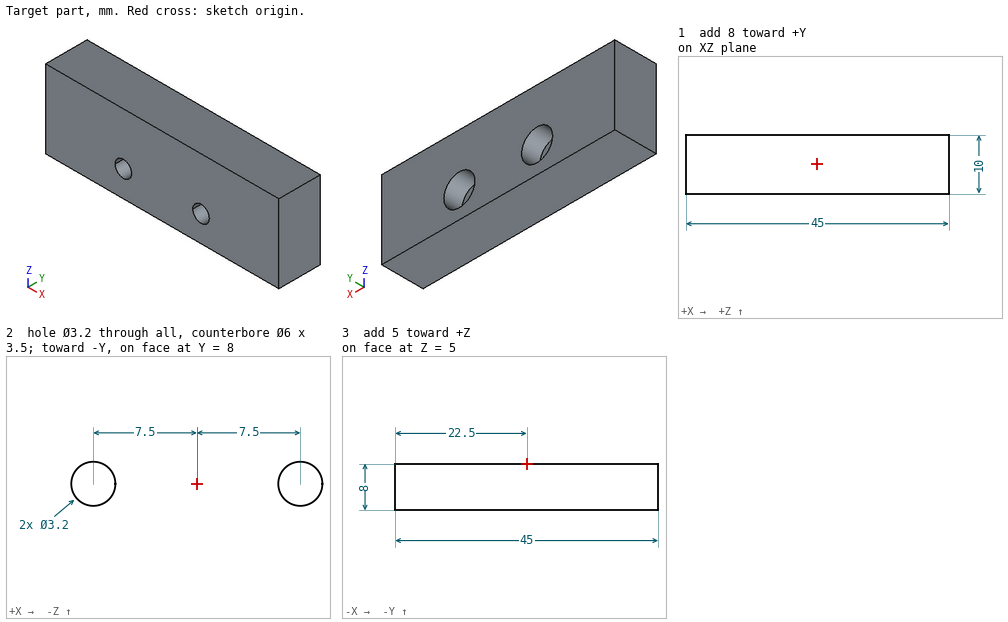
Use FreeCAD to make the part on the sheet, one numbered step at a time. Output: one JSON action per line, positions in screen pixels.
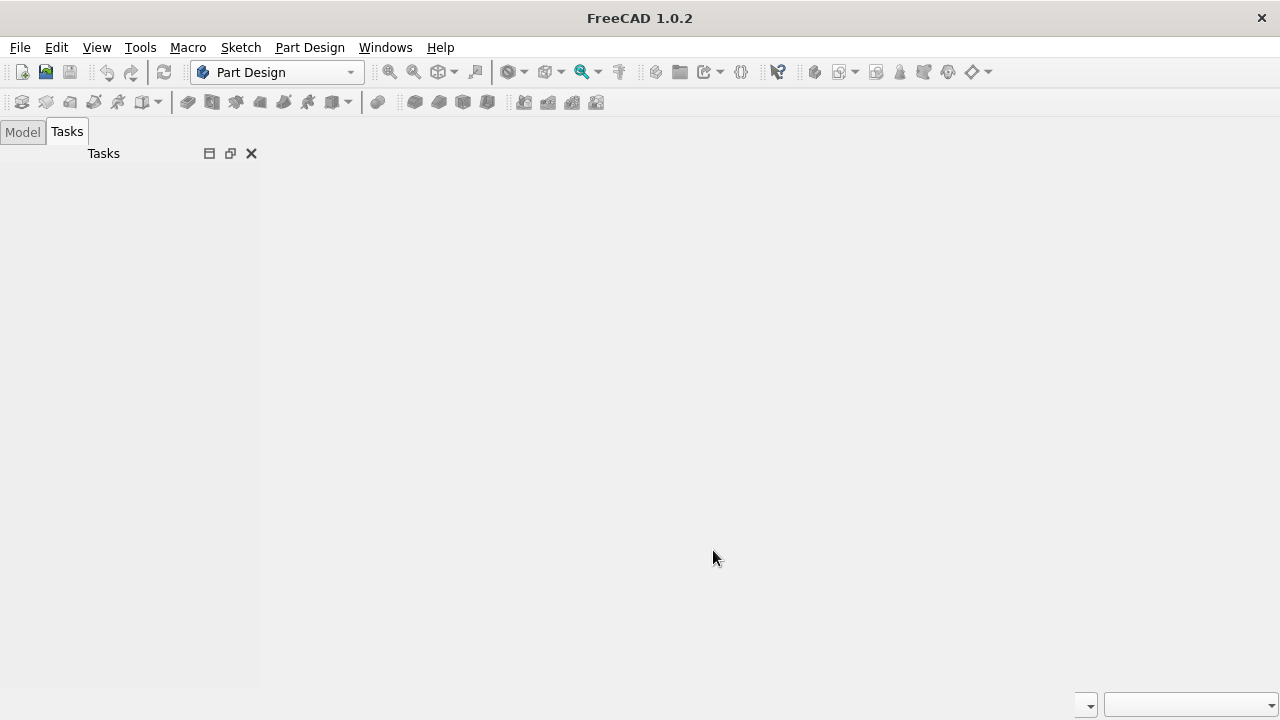
{"action": "left_click", "coordinate": [22, 72]}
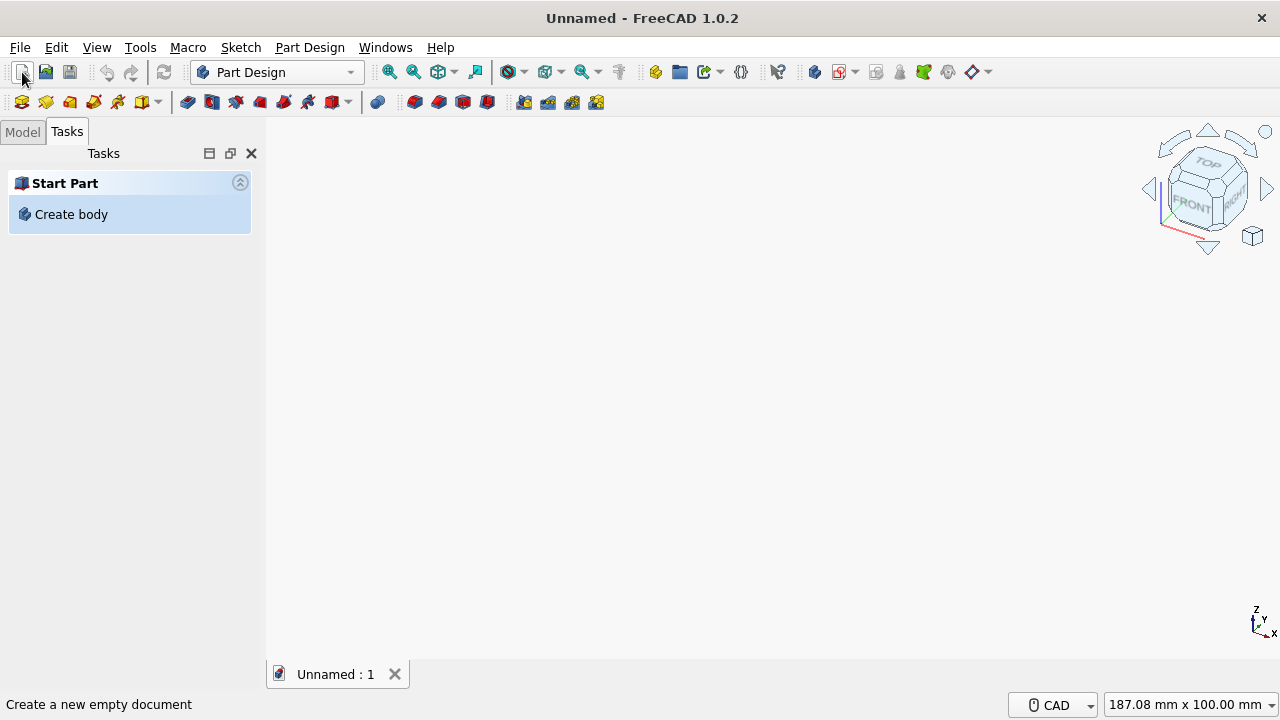
{"action": "left_click", "coordinate": [840, 72]}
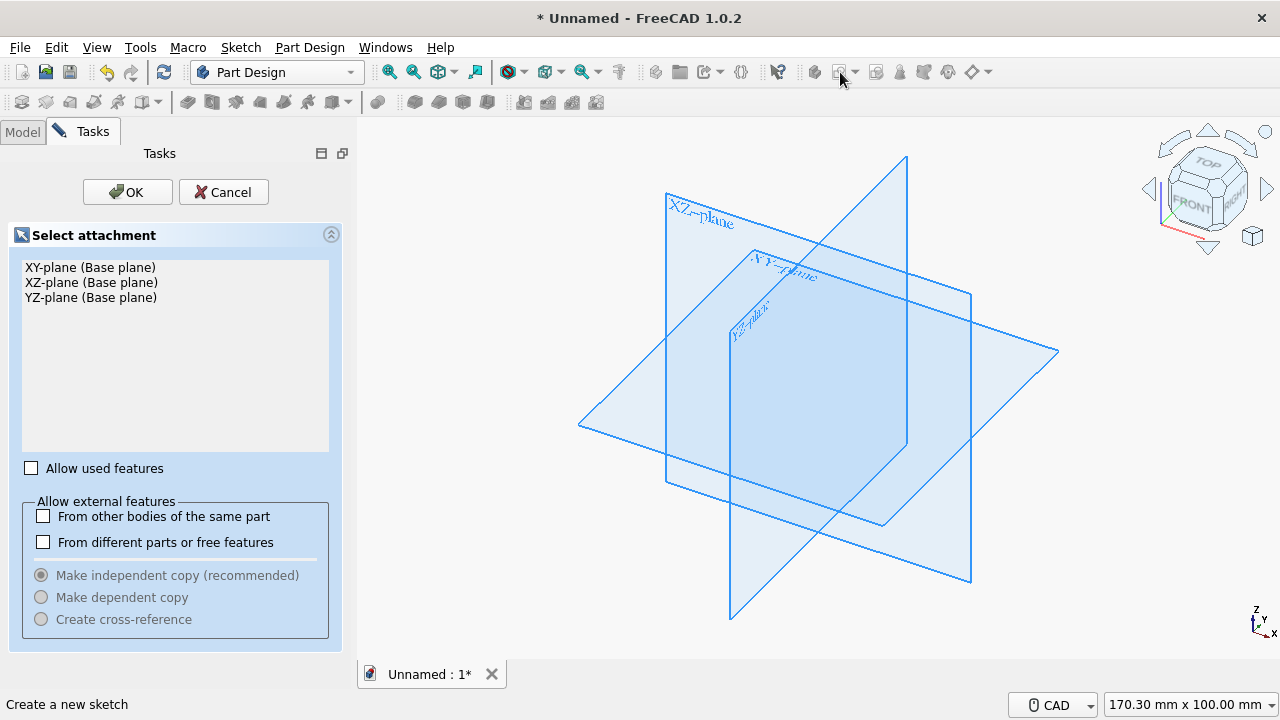
{"action": "left_click", "coordinate": [82, 282]}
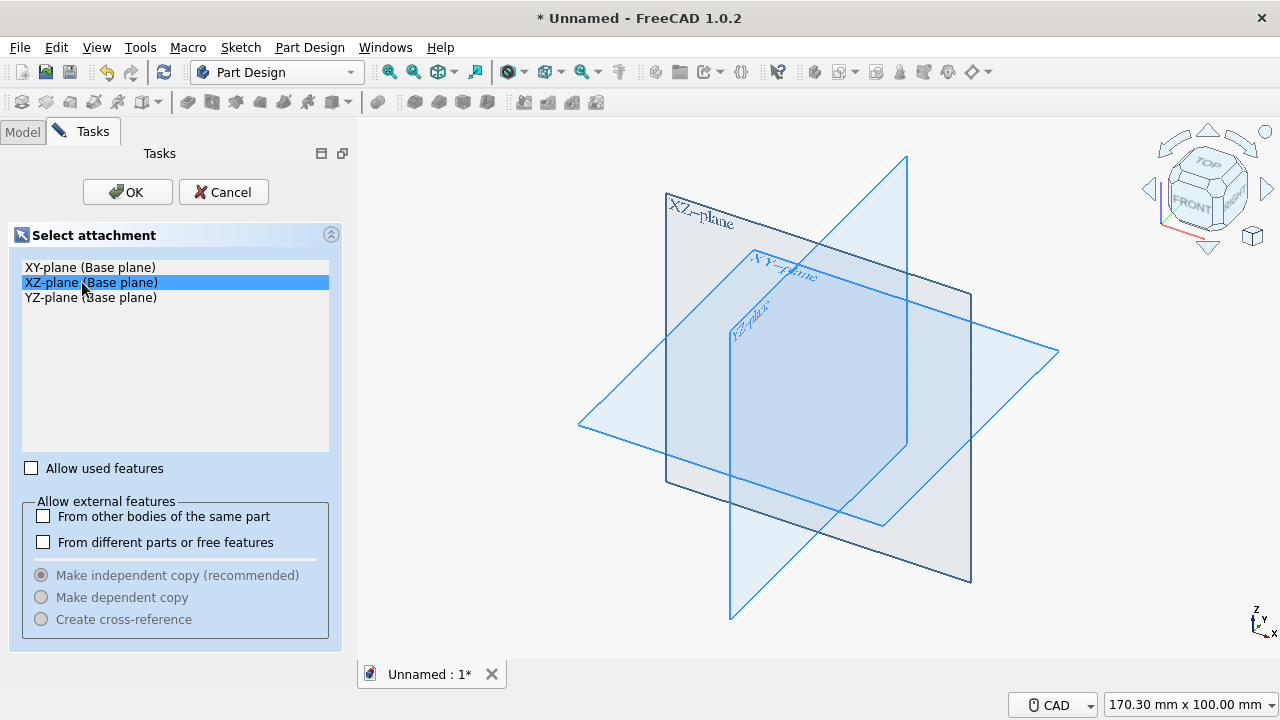
{"action": "left_click", "coordinate": [128, 192]}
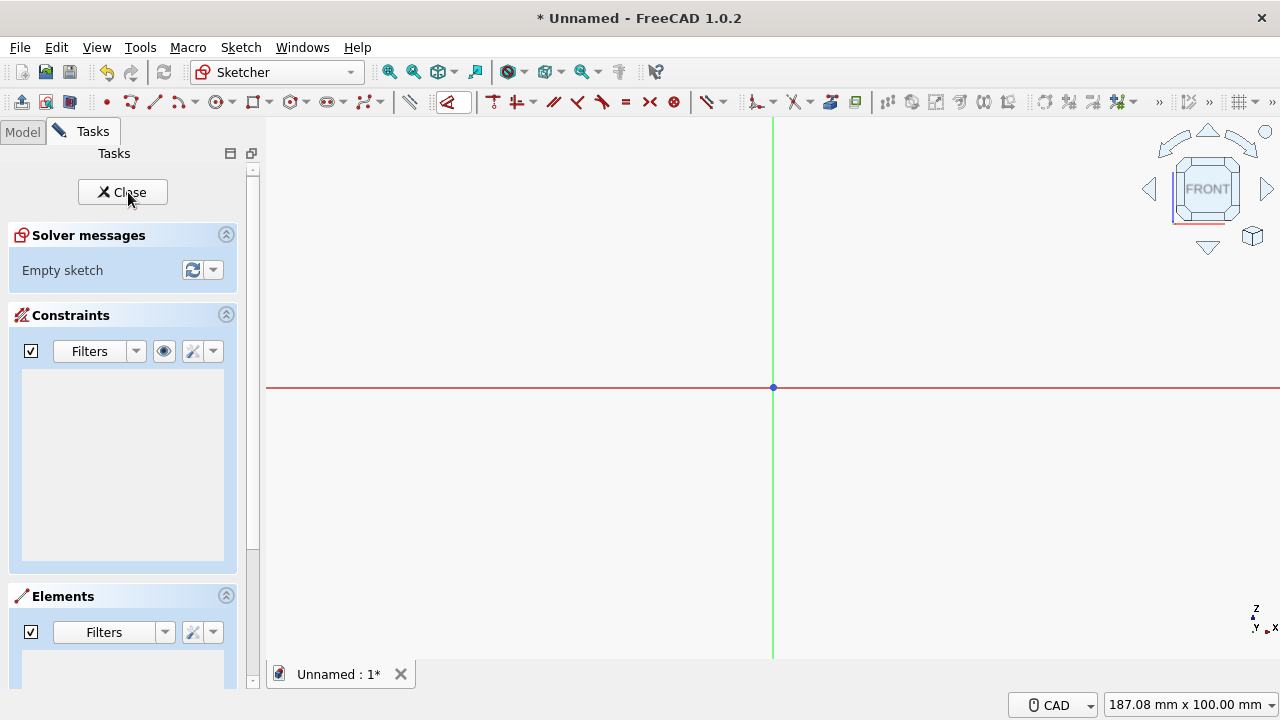
{"action": "scroll", "coordinate": [829, 388], "scroll_direction": "up", "scroll_amount": 4}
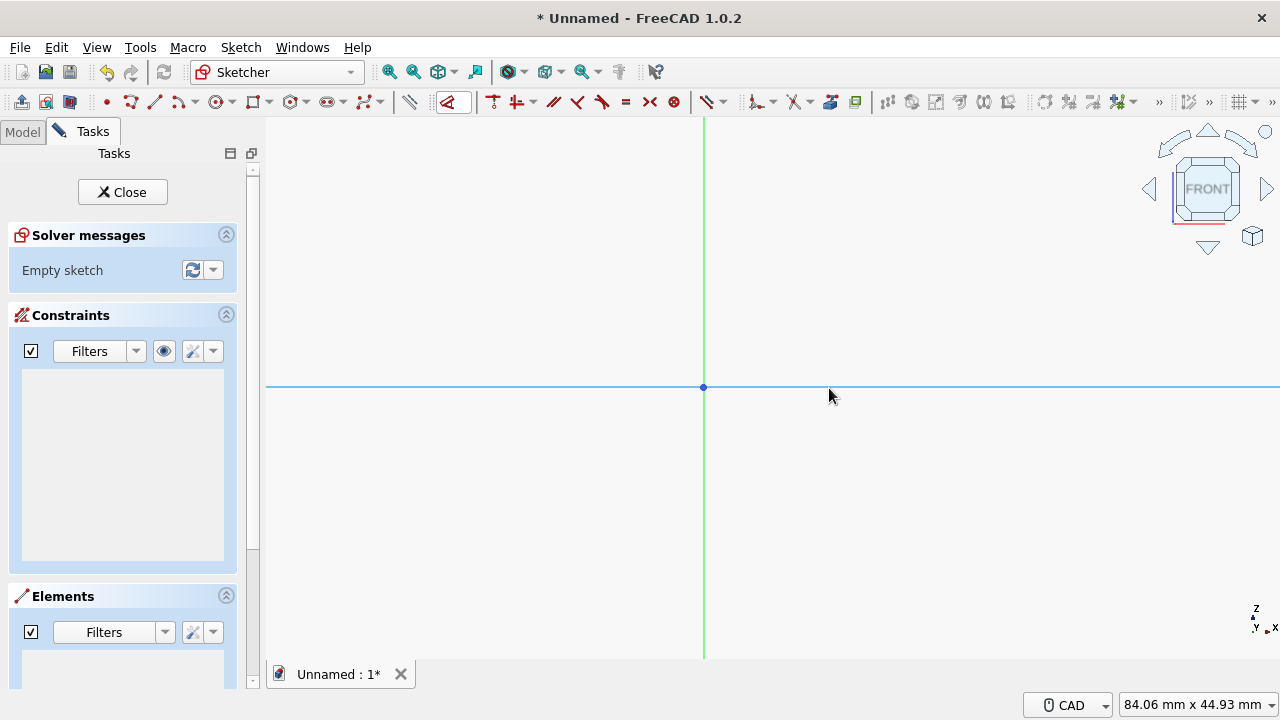
{"action": "left_click", "coordinate": [272, 102]}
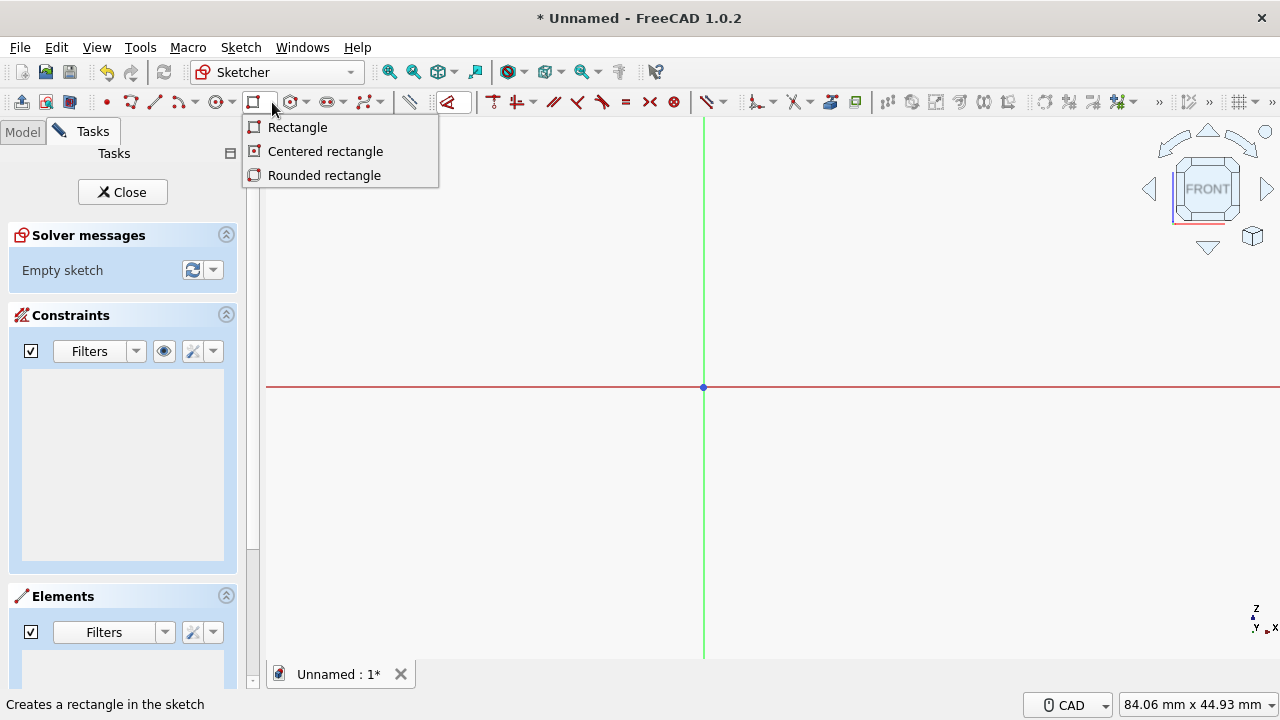
{"action": "left_click", "coordinate": [340, 151]}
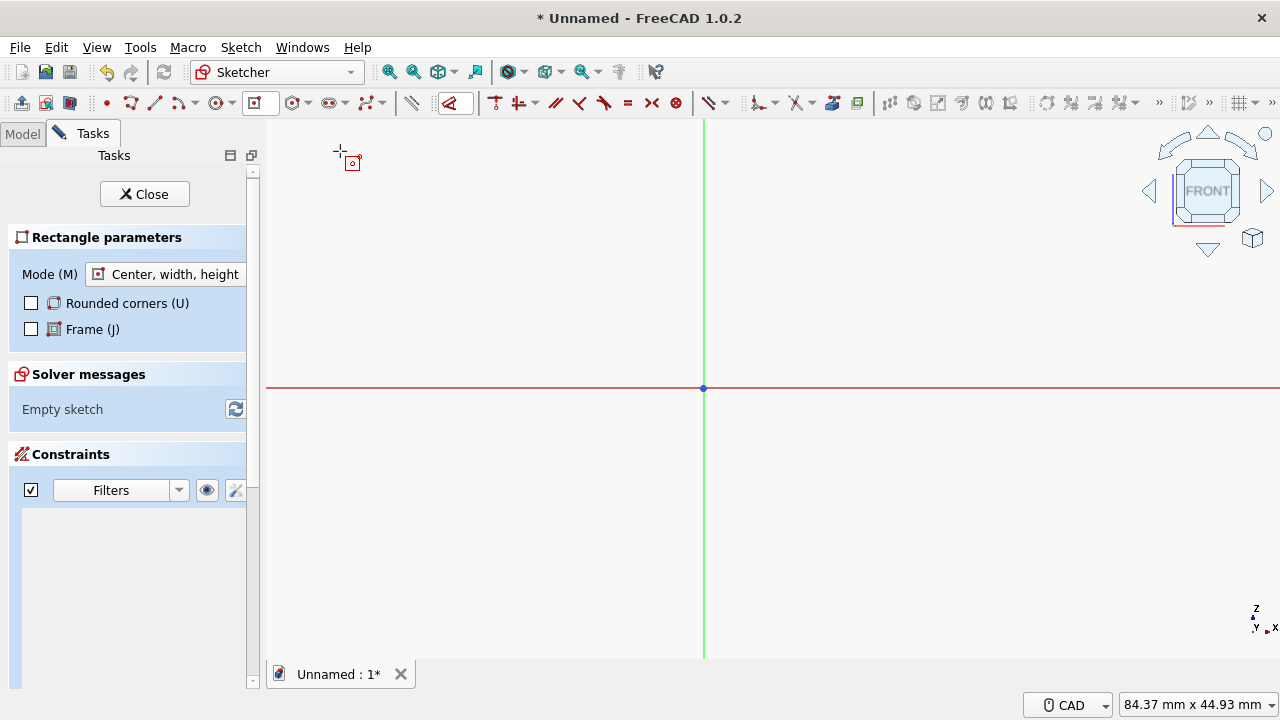
{"action": "left_click", "coordinate": [704, 388]}
{"action": "left_click", "coordinate": [974, 328]}
{"action": "key", "text": "Escape"}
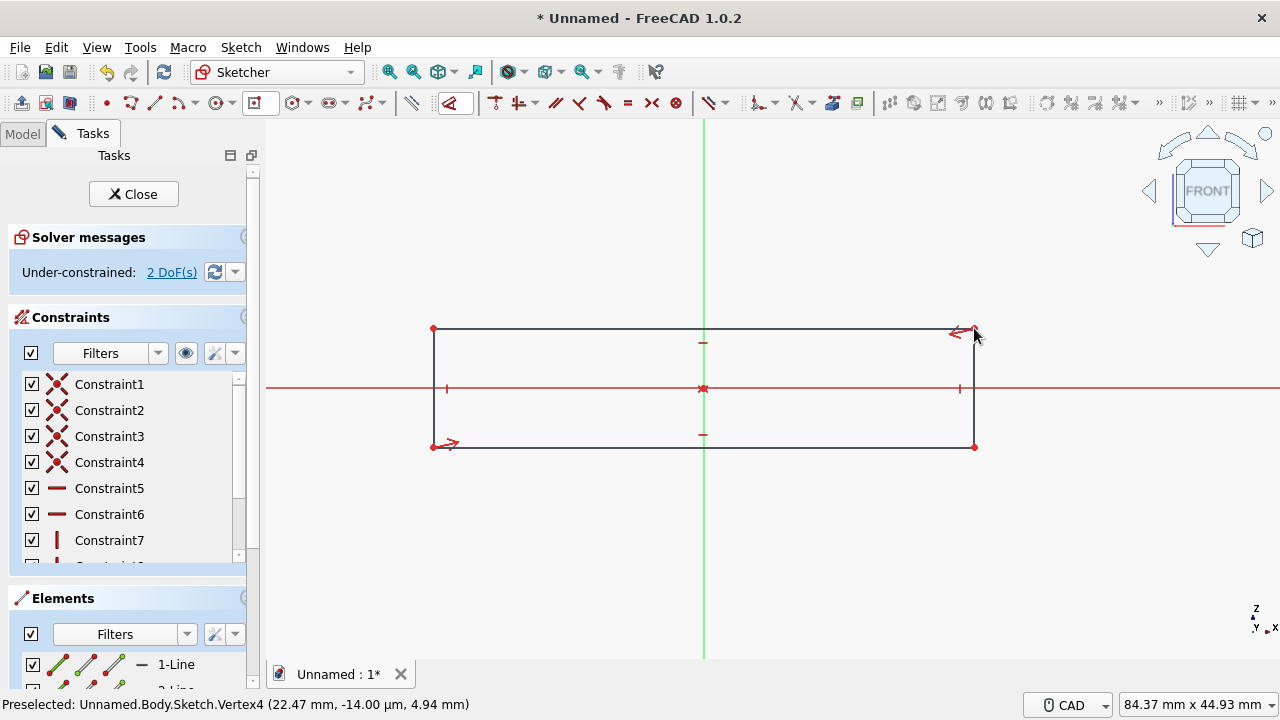
{"action": "left_click", "coordinate": [450, 104]}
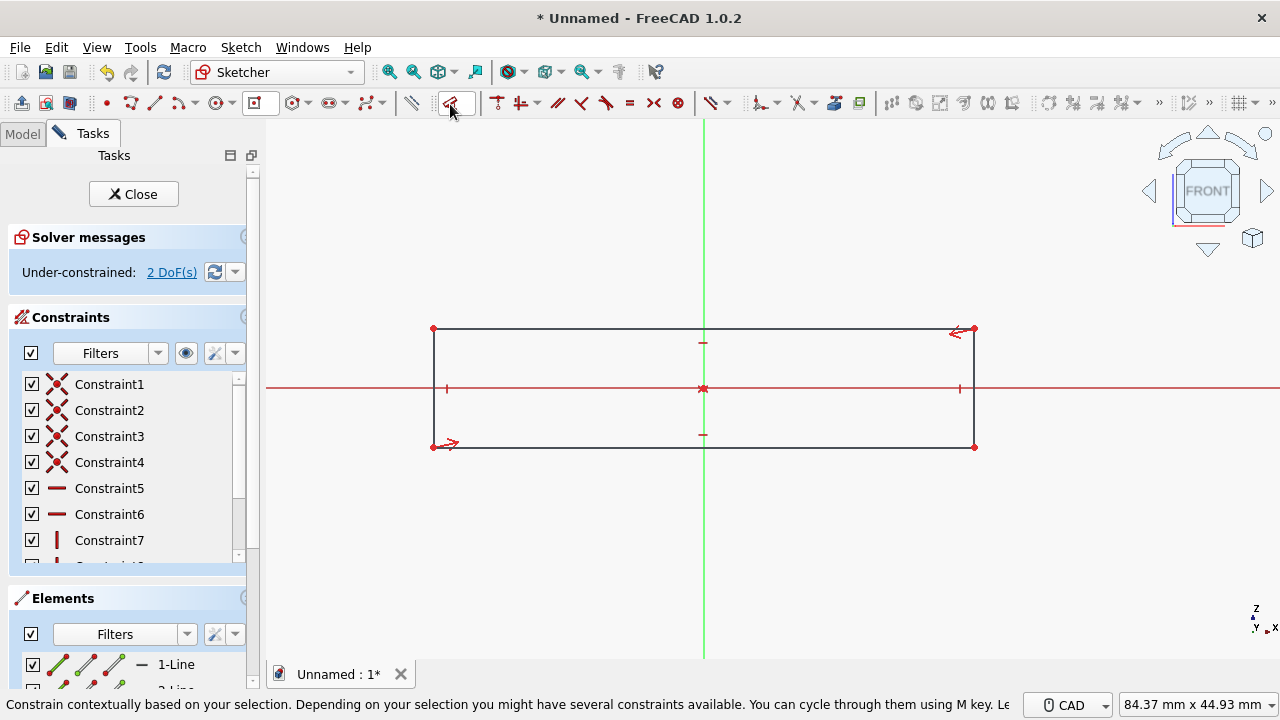
{"action": "left_click", "coordinate": [596, 448]}
{"action": "left_click", "coordinate": [580, 482]}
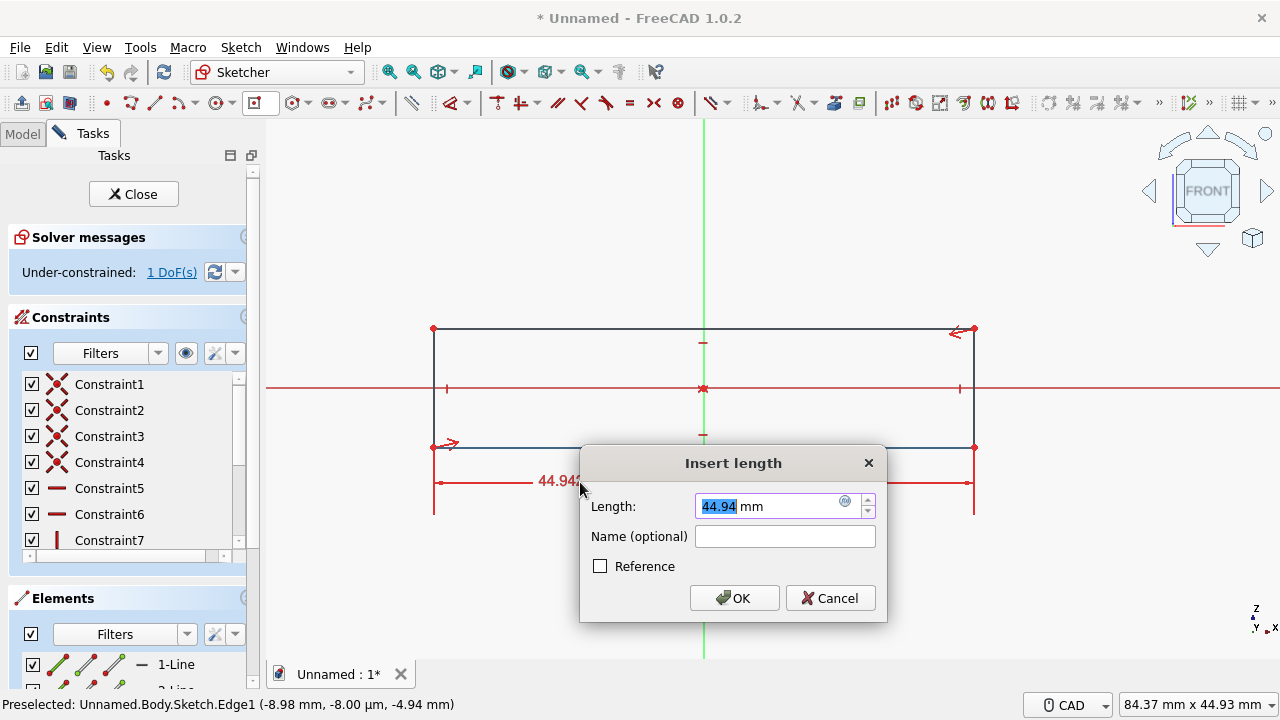
{"action": "type", "text": "45"}
{"action": "key", "text": "Return"}